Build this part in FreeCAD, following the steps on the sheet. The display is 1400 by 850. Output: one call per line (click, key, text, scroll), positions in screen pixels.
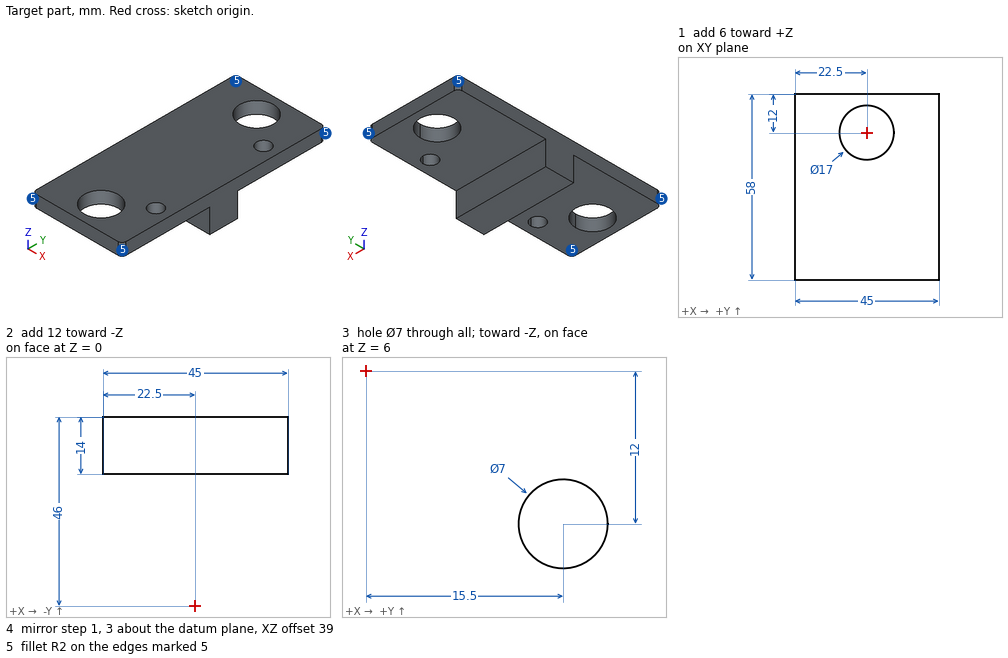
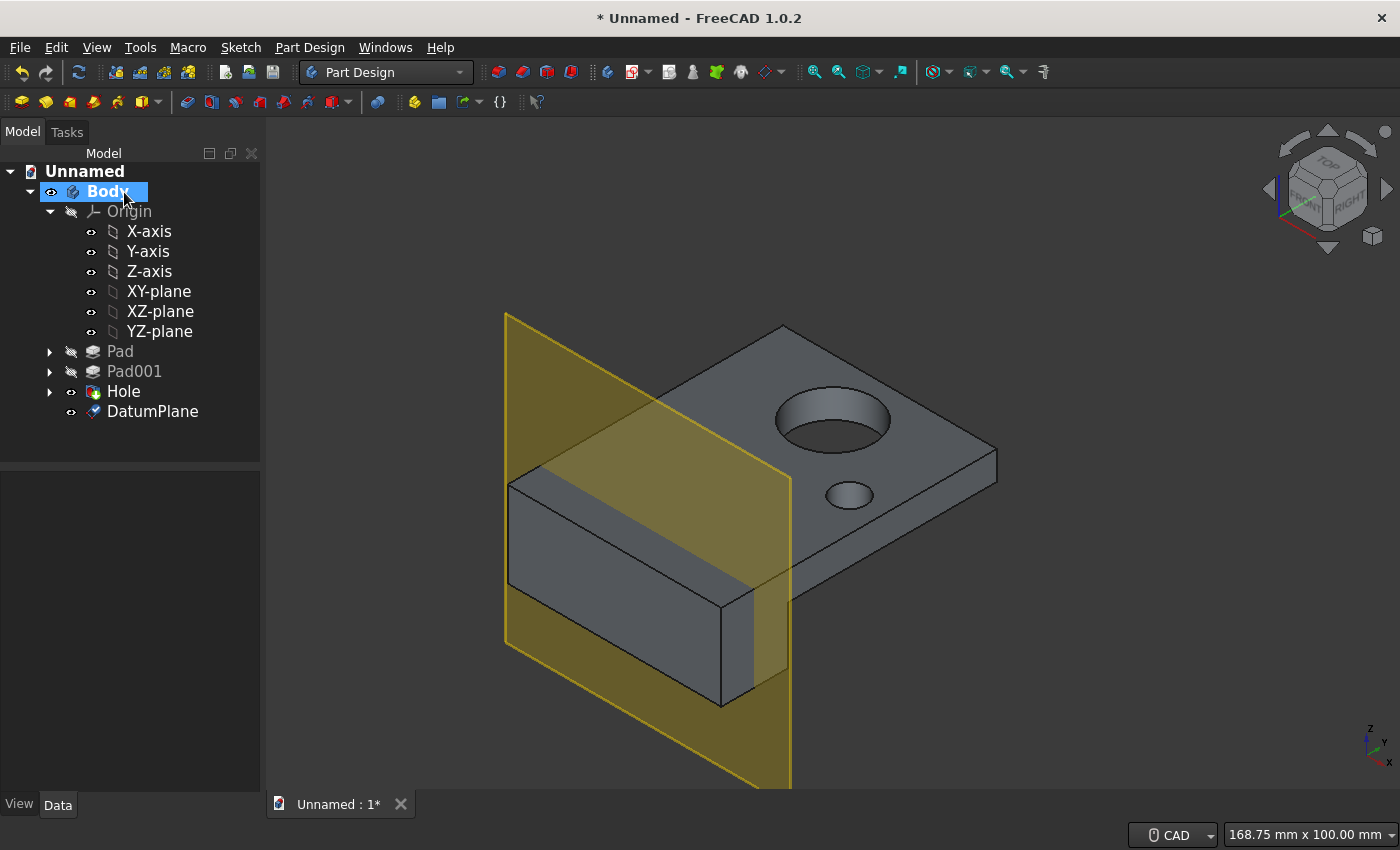
click(116, 352)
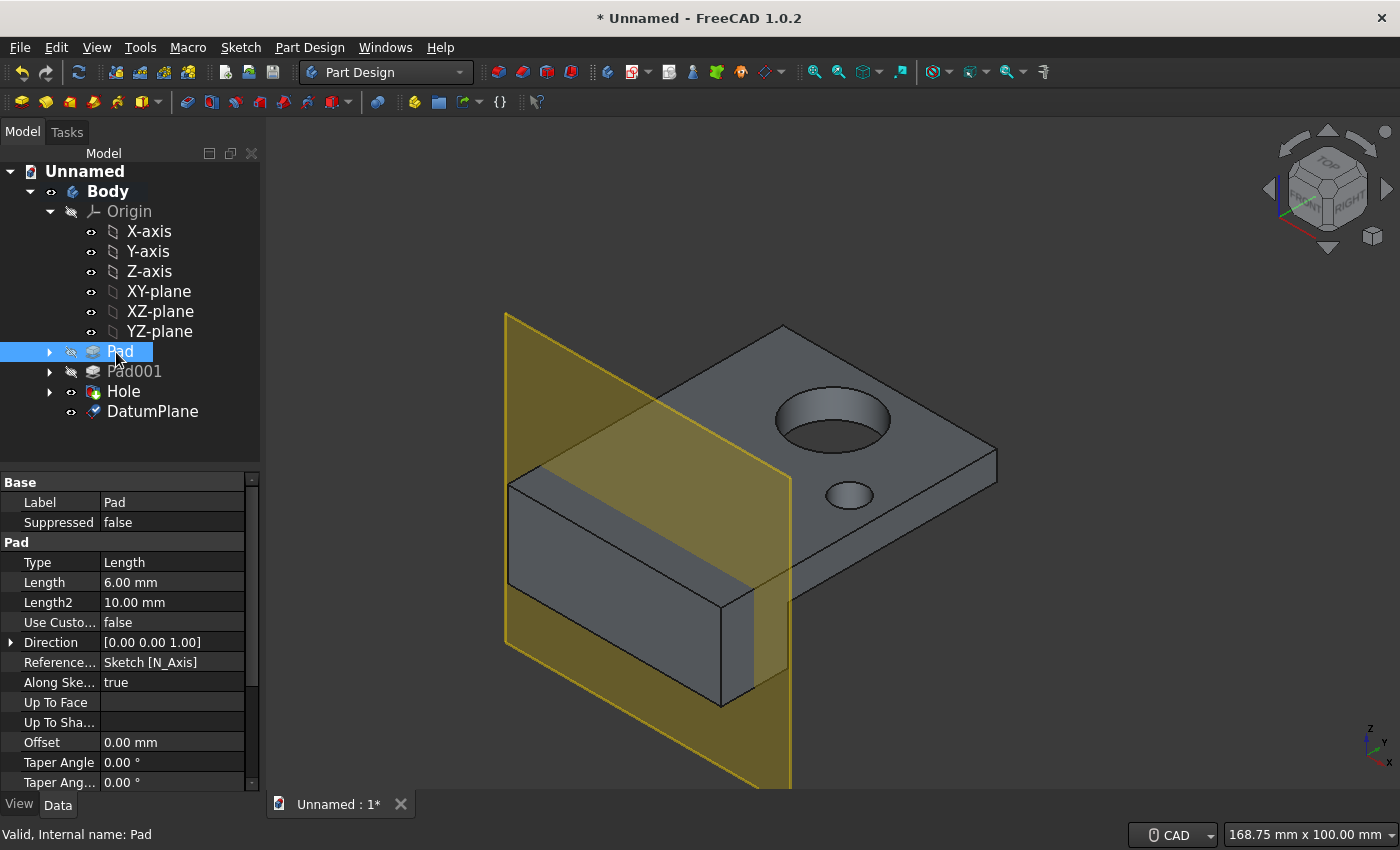
click(116, 392, ctrl)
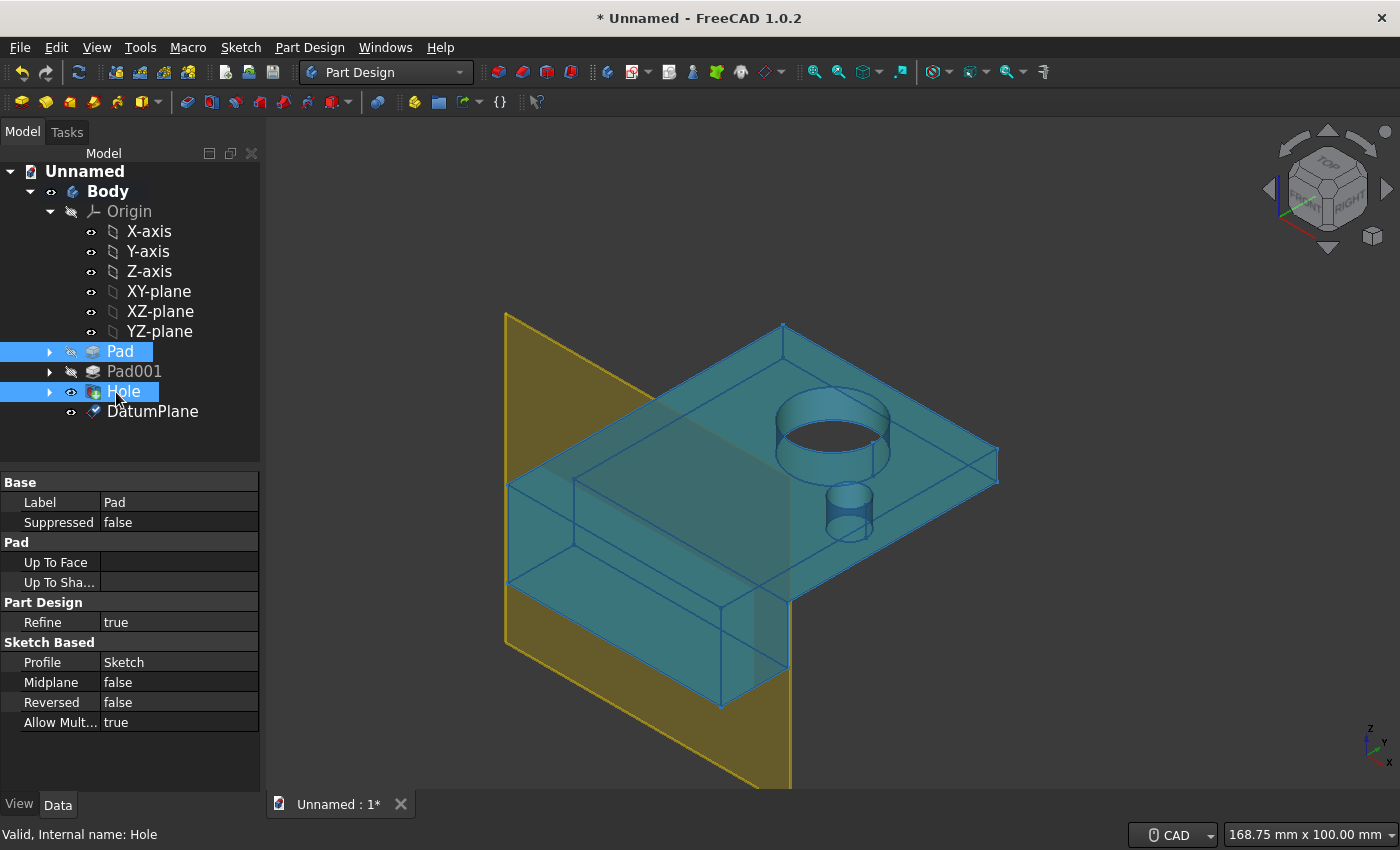
click(116, 72)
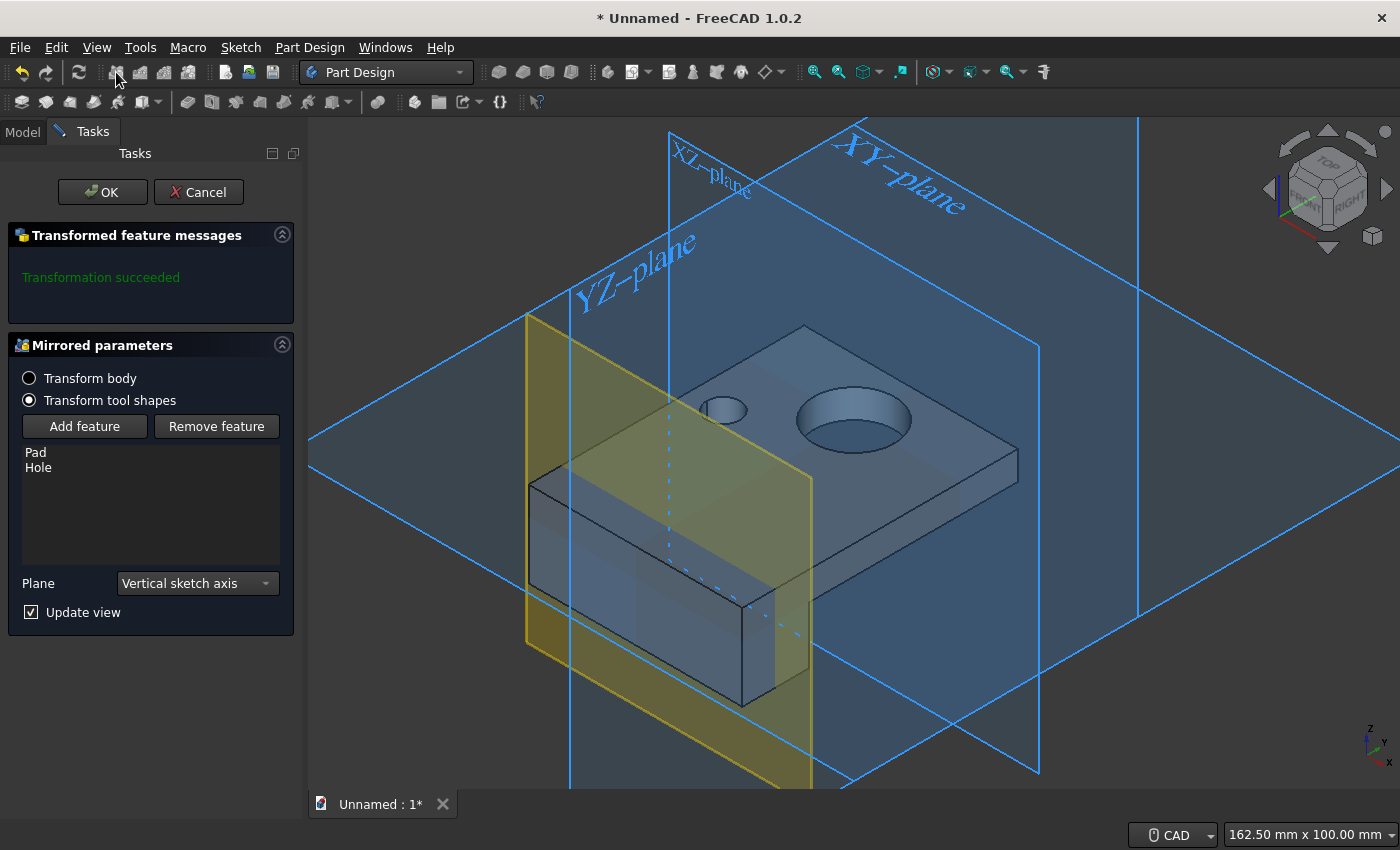
click(198, 584)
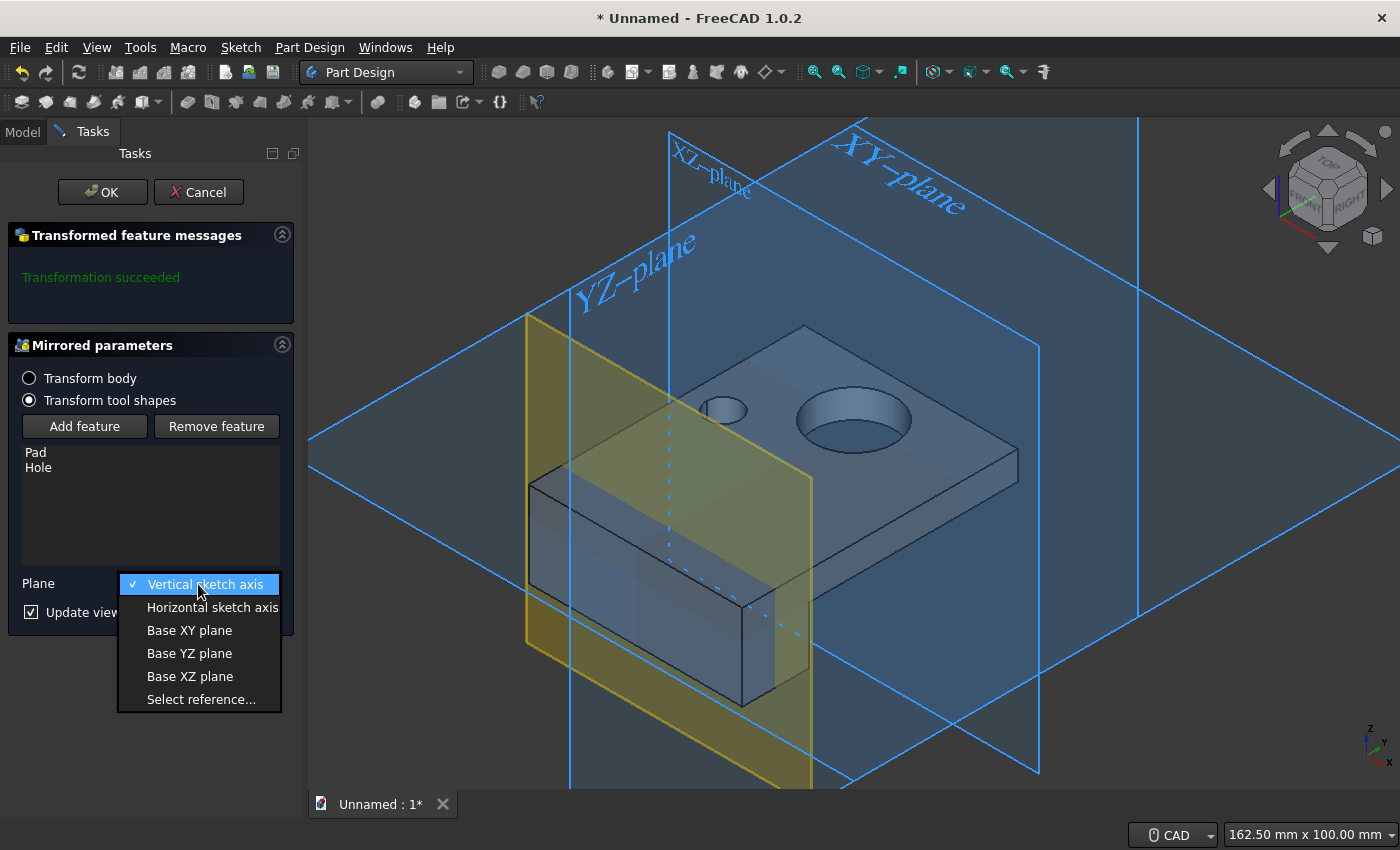
click(198, 700)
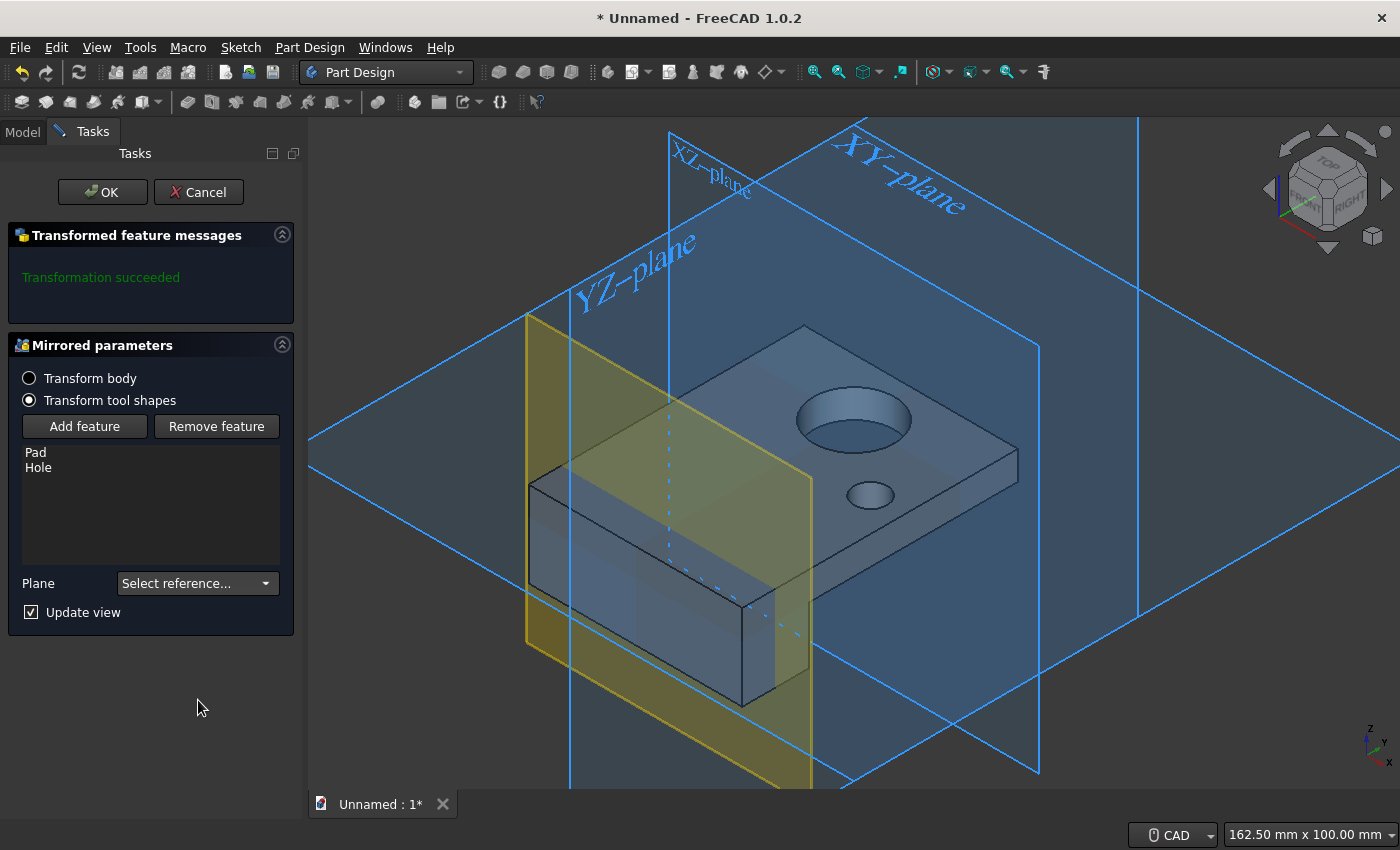
click(23, 131)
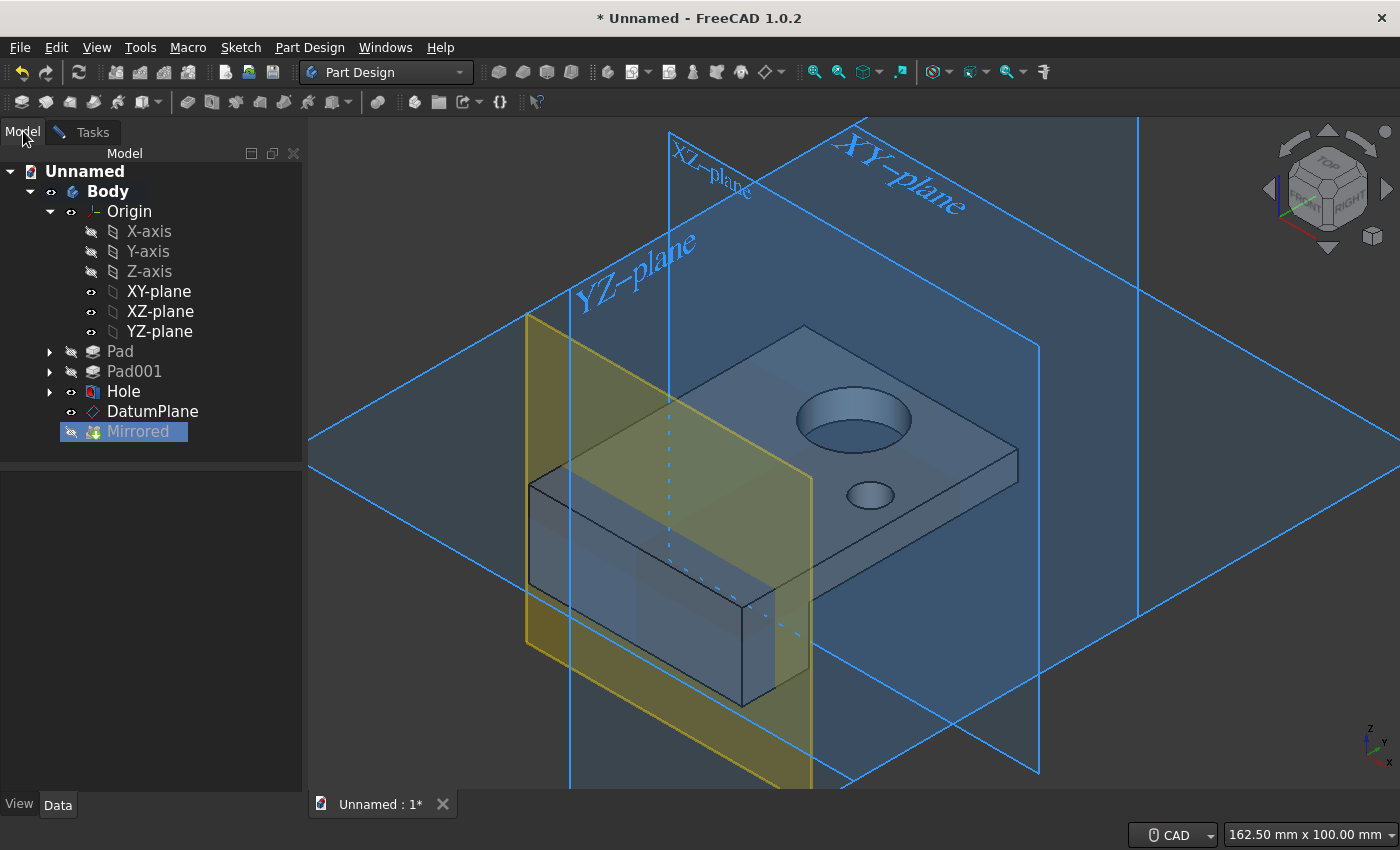
click(116, 412)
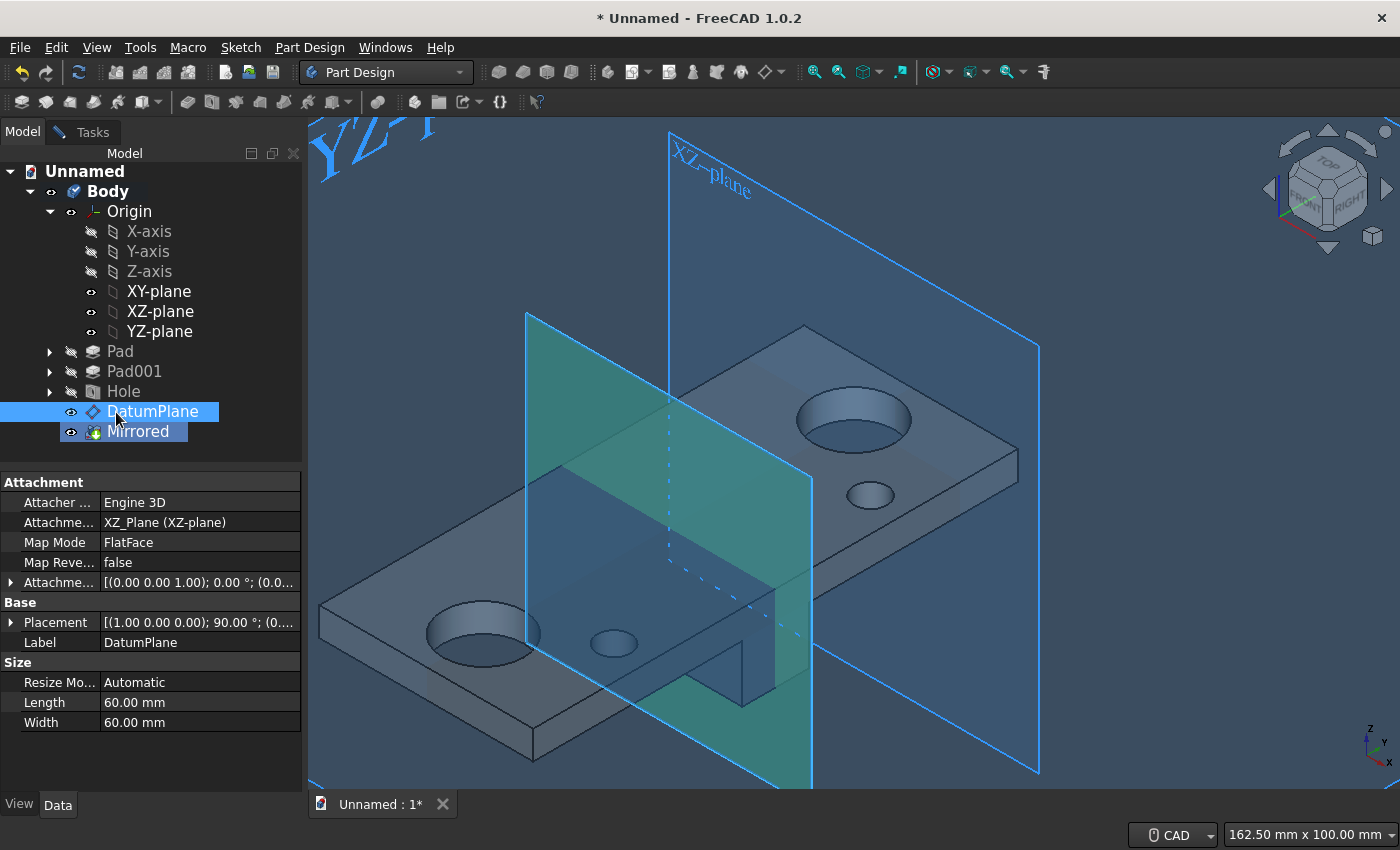
click(84, 131)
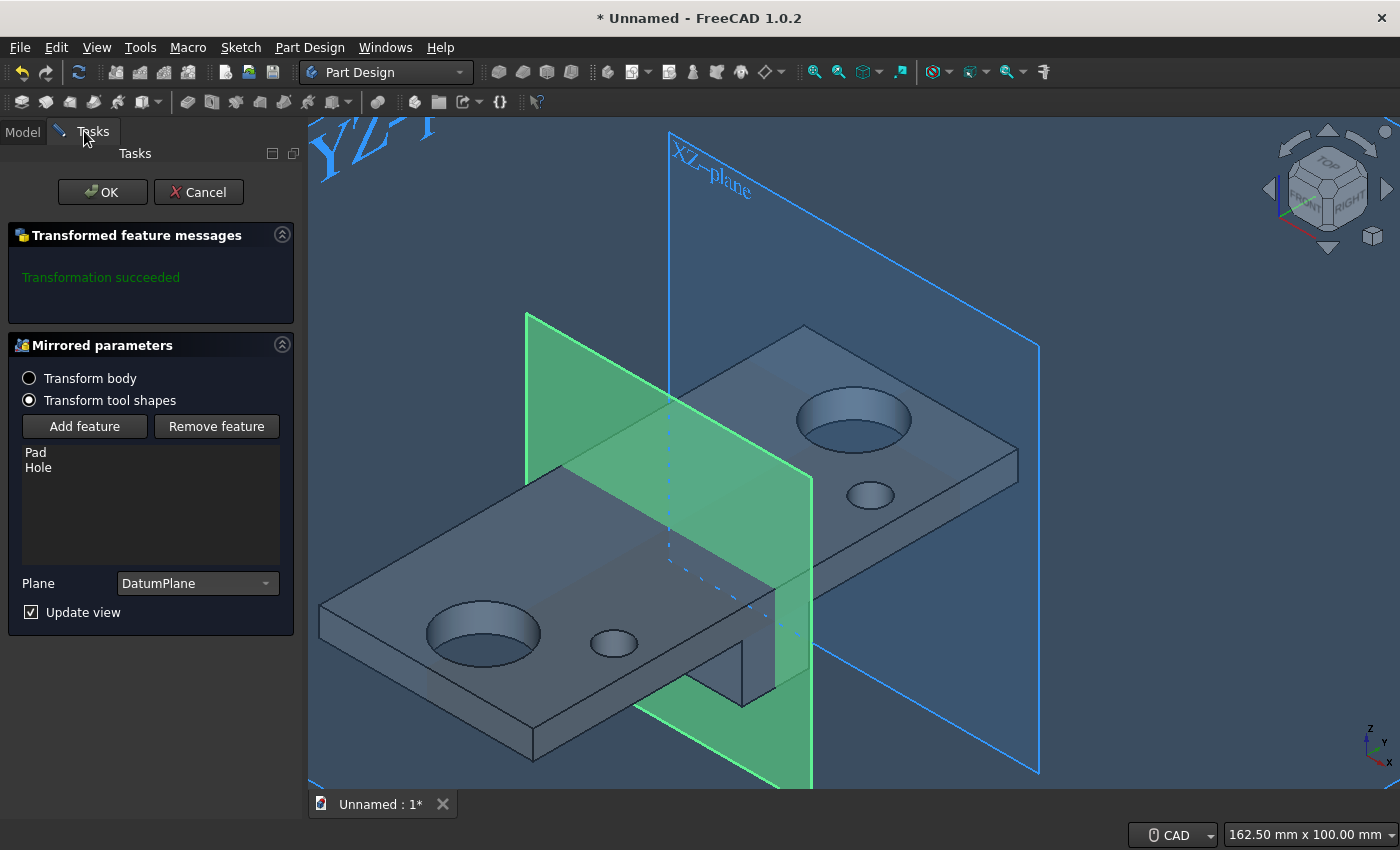
click(103, 192)